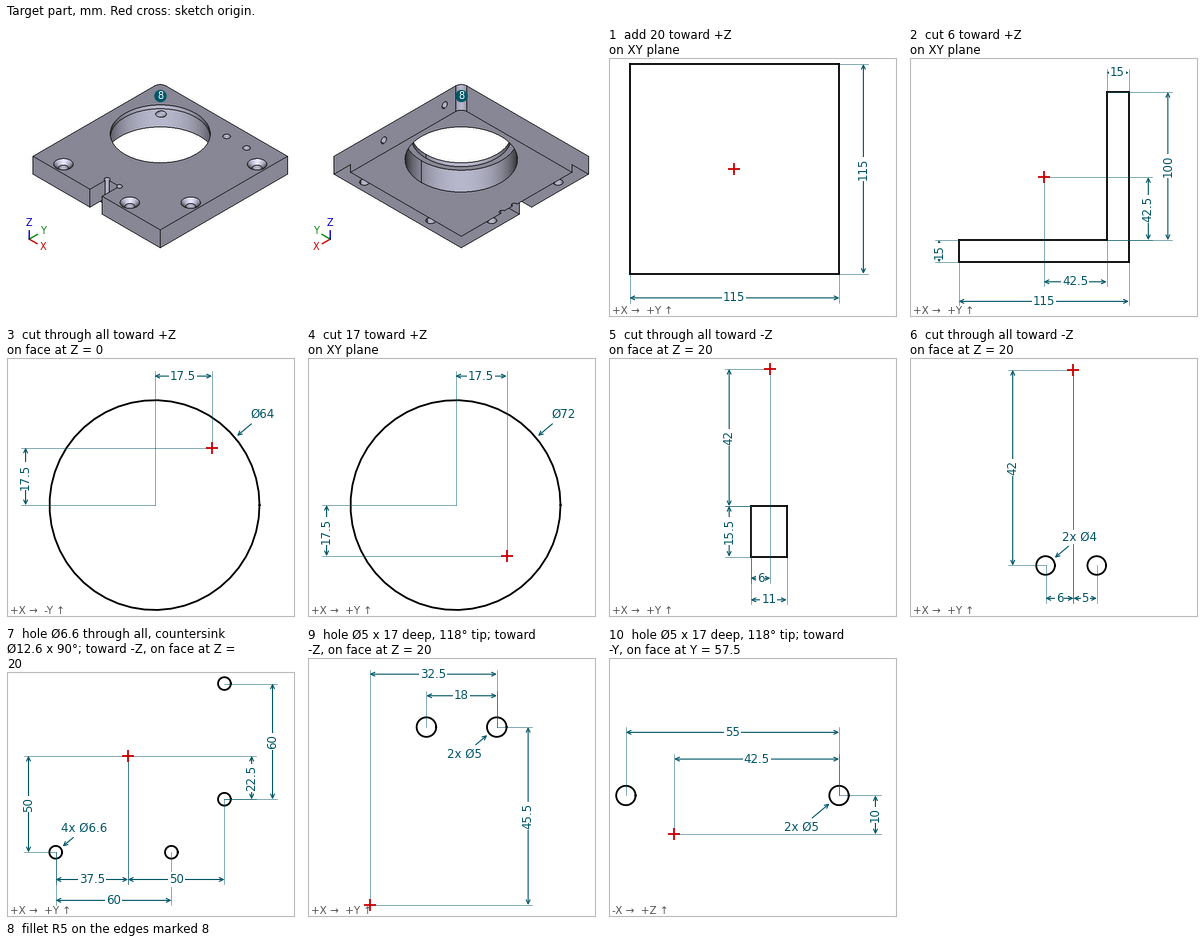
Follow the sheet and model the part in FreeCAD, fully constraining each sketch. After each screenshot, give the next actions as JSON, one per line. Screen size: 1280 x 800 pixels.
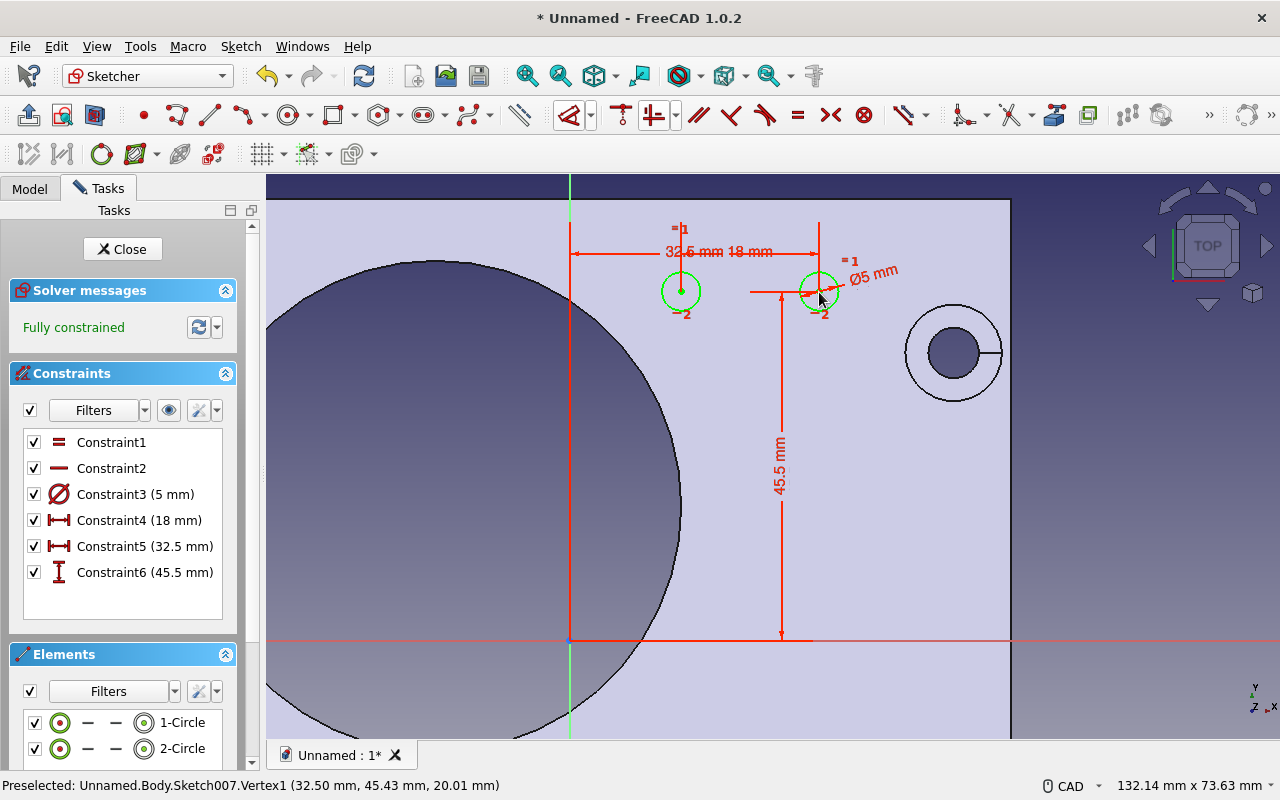
{"action": "left_click", "coordinate": [123, 249]}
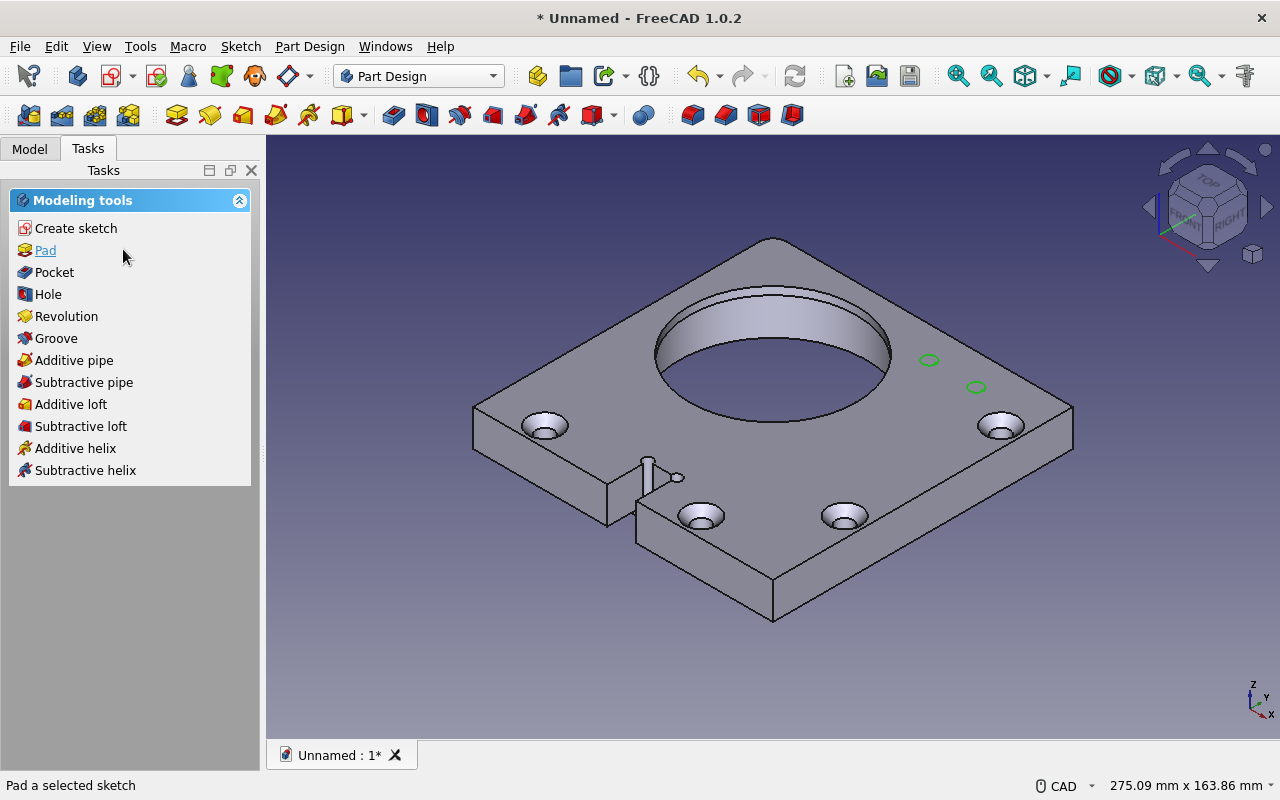
{"action": "left_click", "coordinate": [427, 116]}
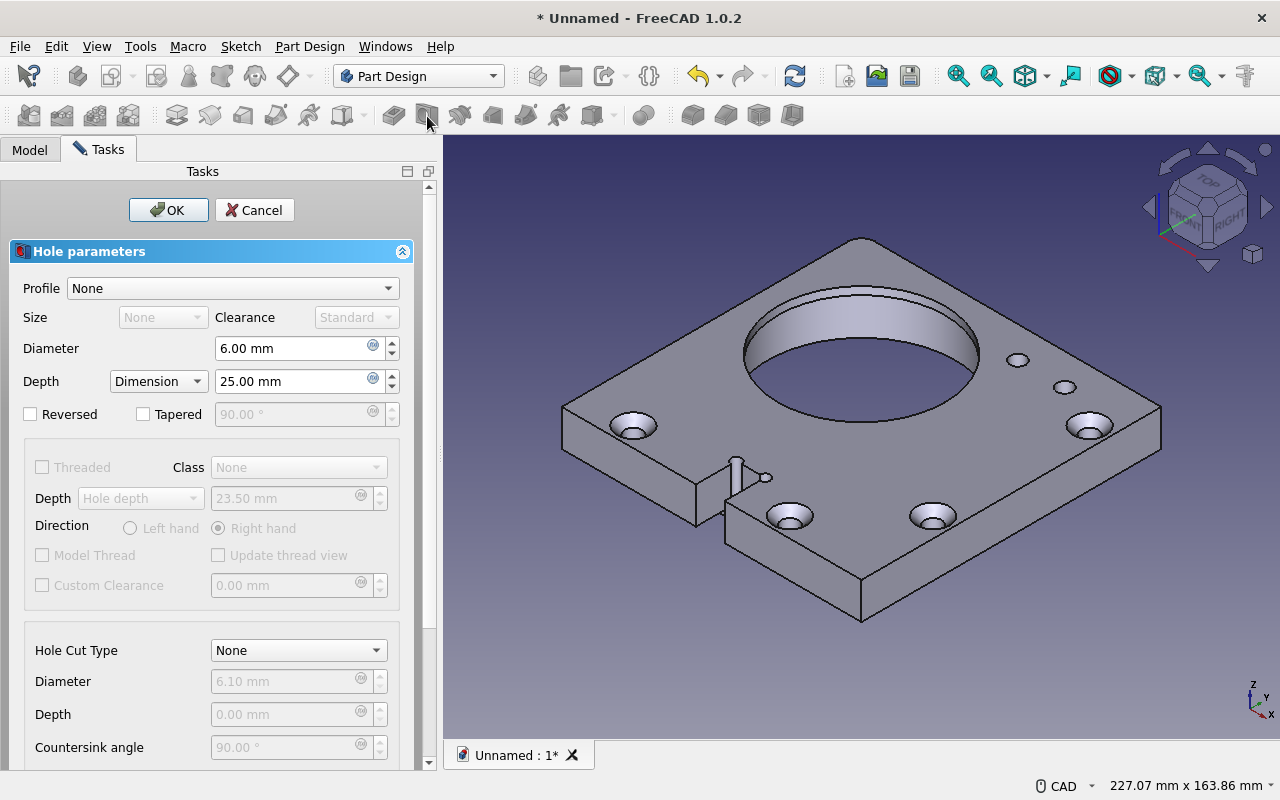
{"action": "triple_click", "coordinate": [300, 348]}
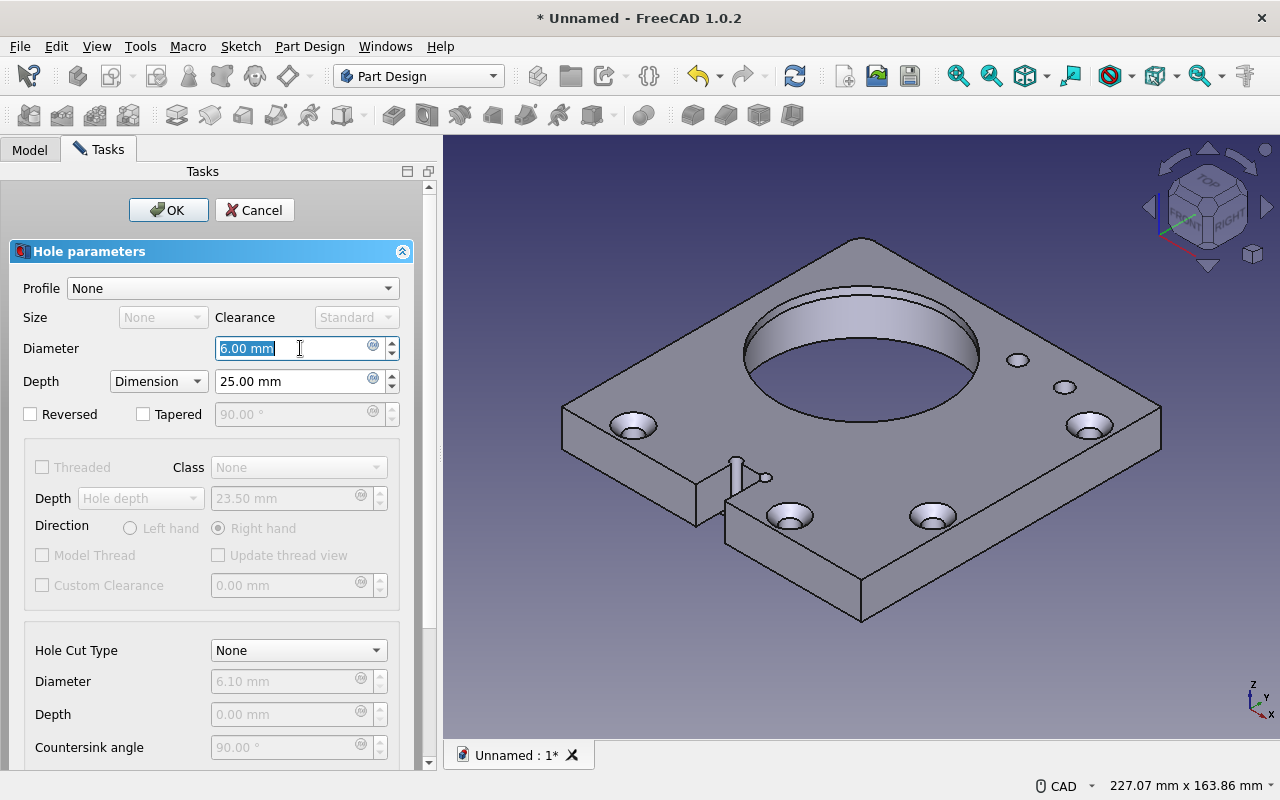
{"action": "type", "text": "5"}
{"action": "key", "text": "Tab"}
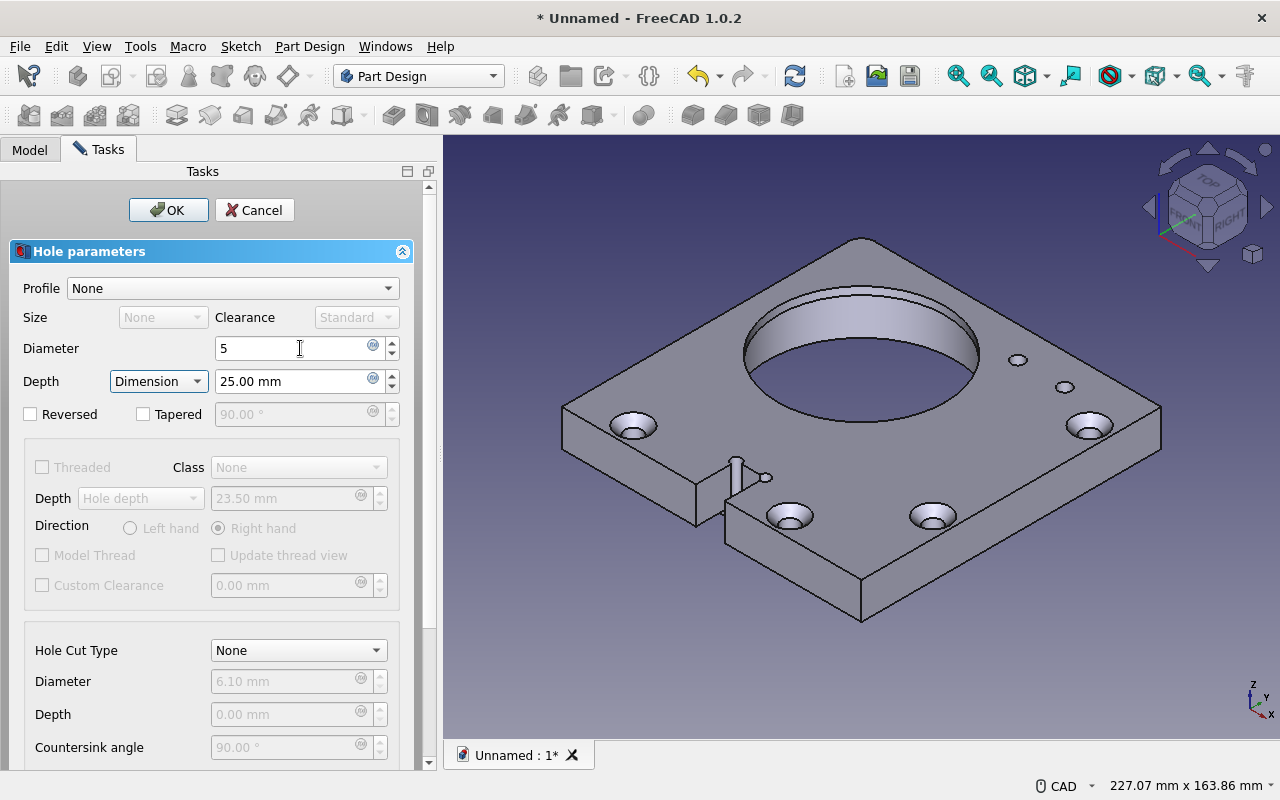
{"action": "triple_click", "coordinate": [300, 382]}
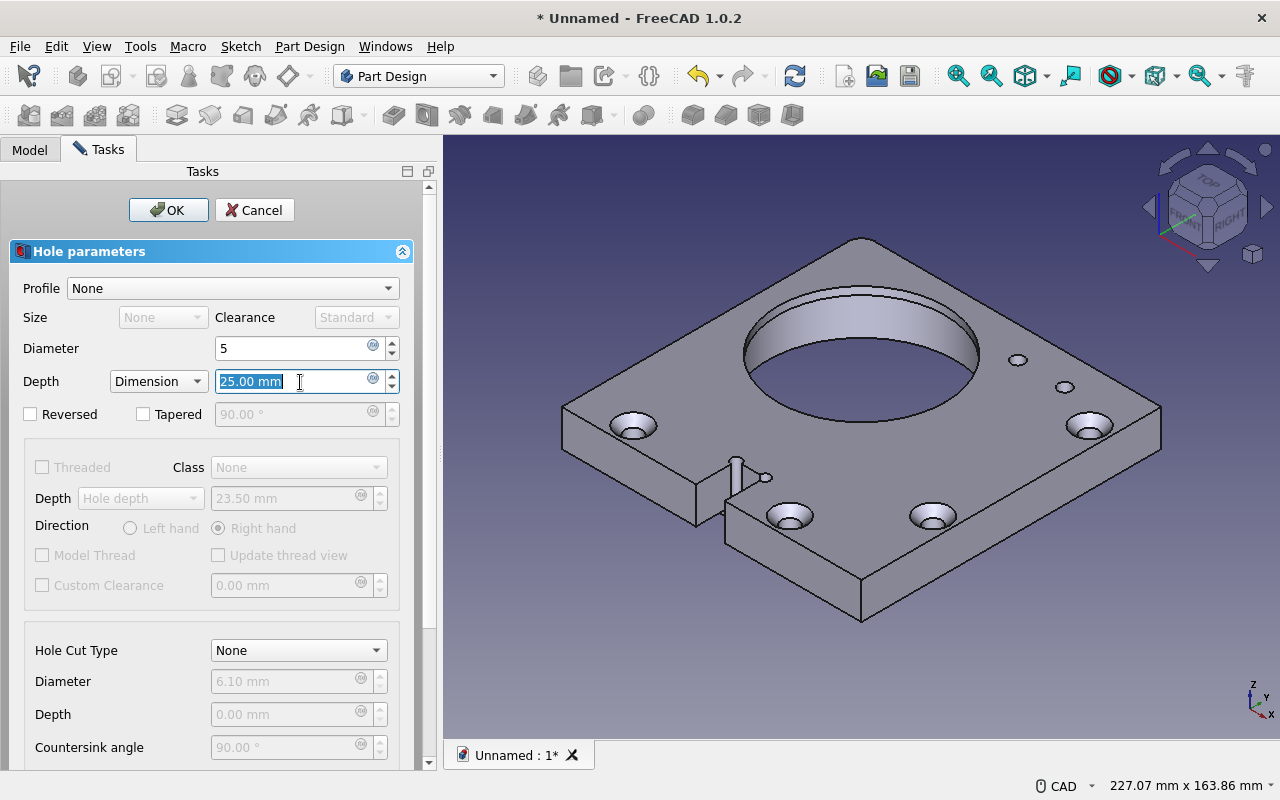
{"action": "type", "text": "17"}
{"action": "key", "text": "Tab"}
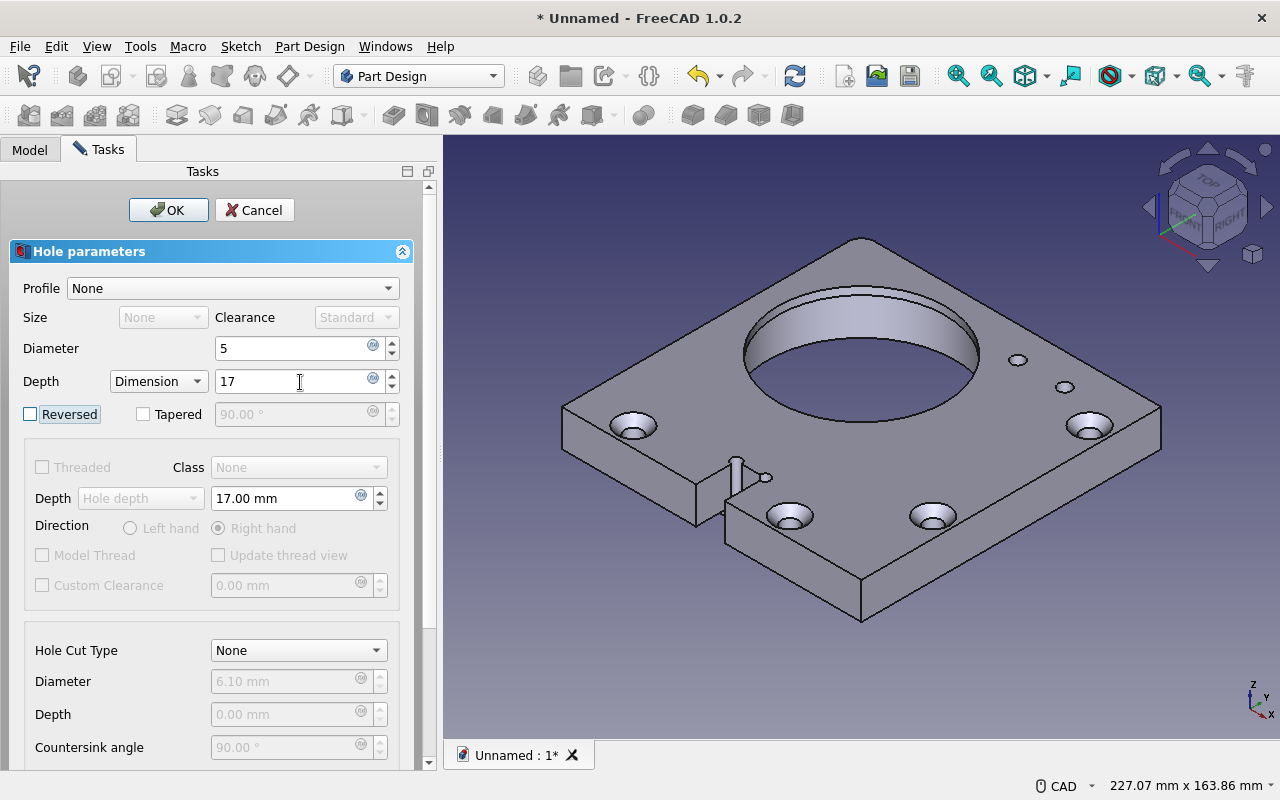
{"action": "left_click", "coordinate": [169, 210]}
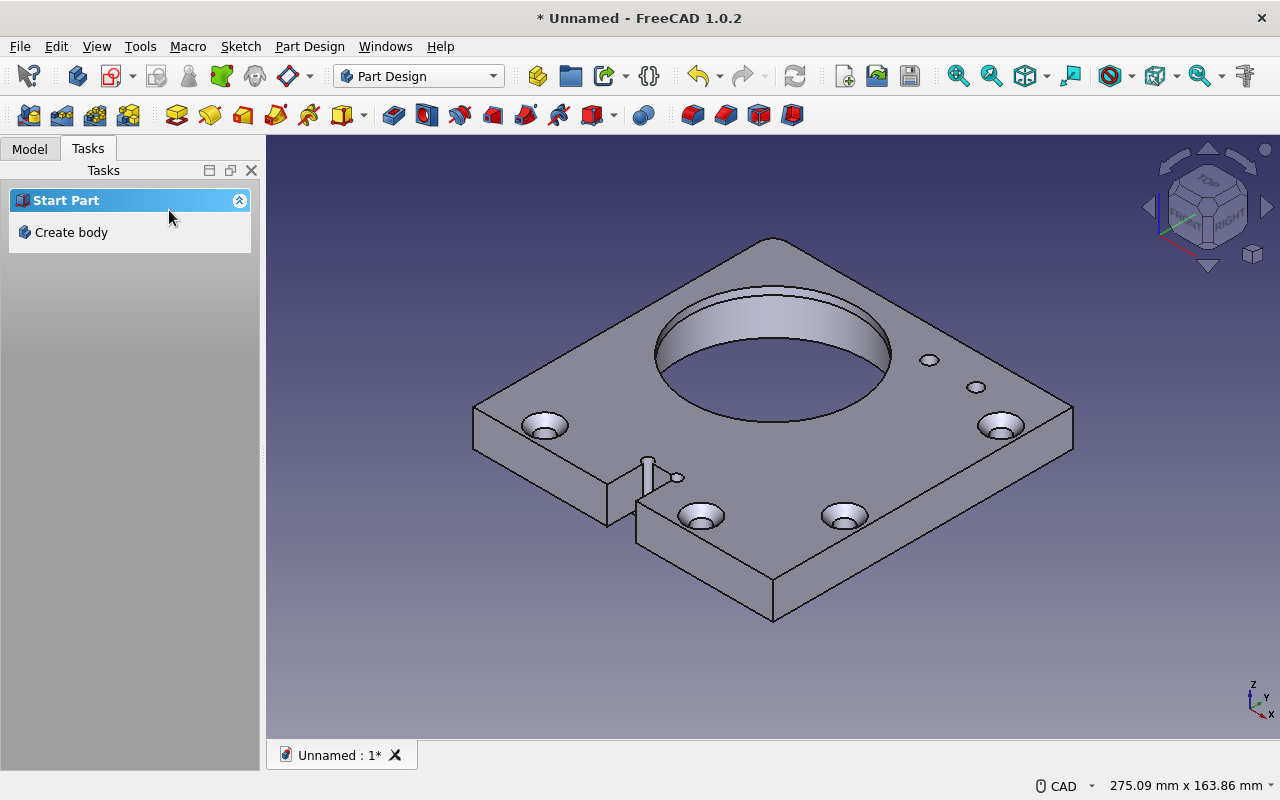
{"action": "key", "text": "4"}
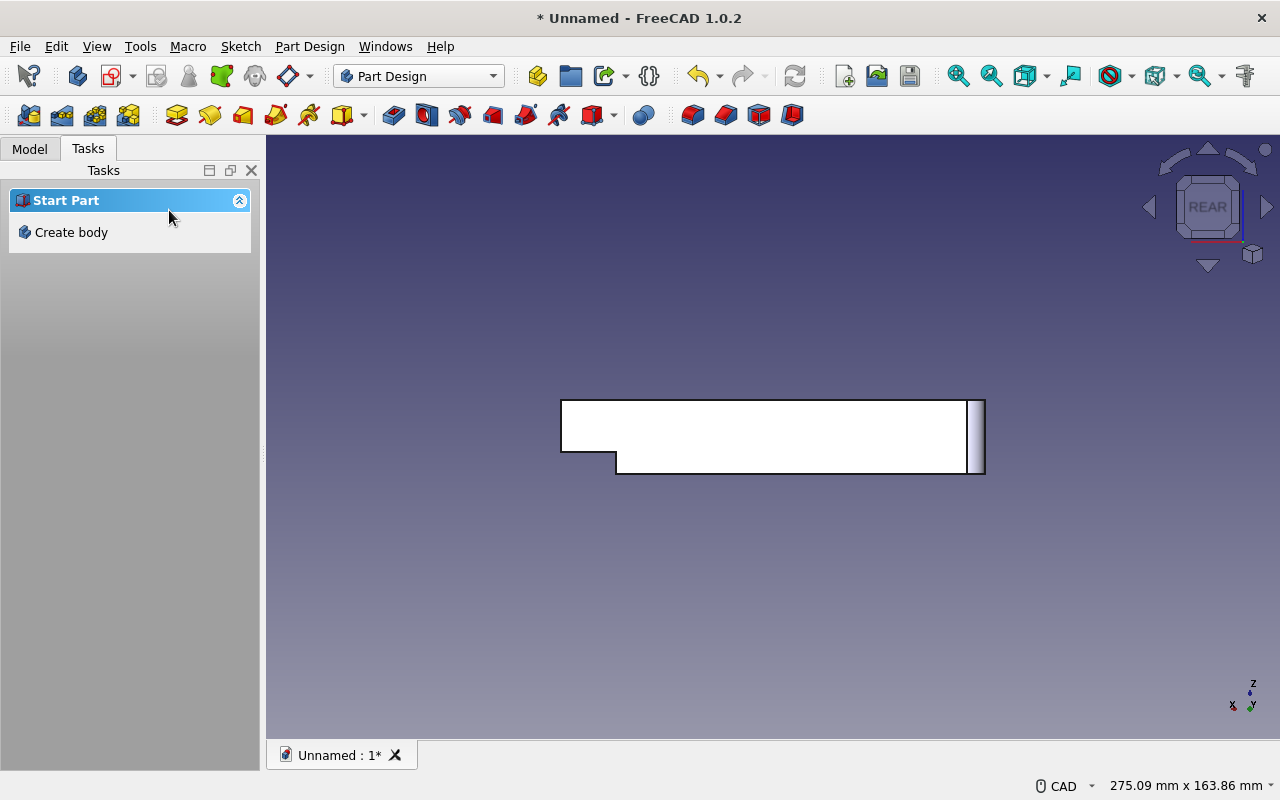
{"action": "key", "text": "v f"}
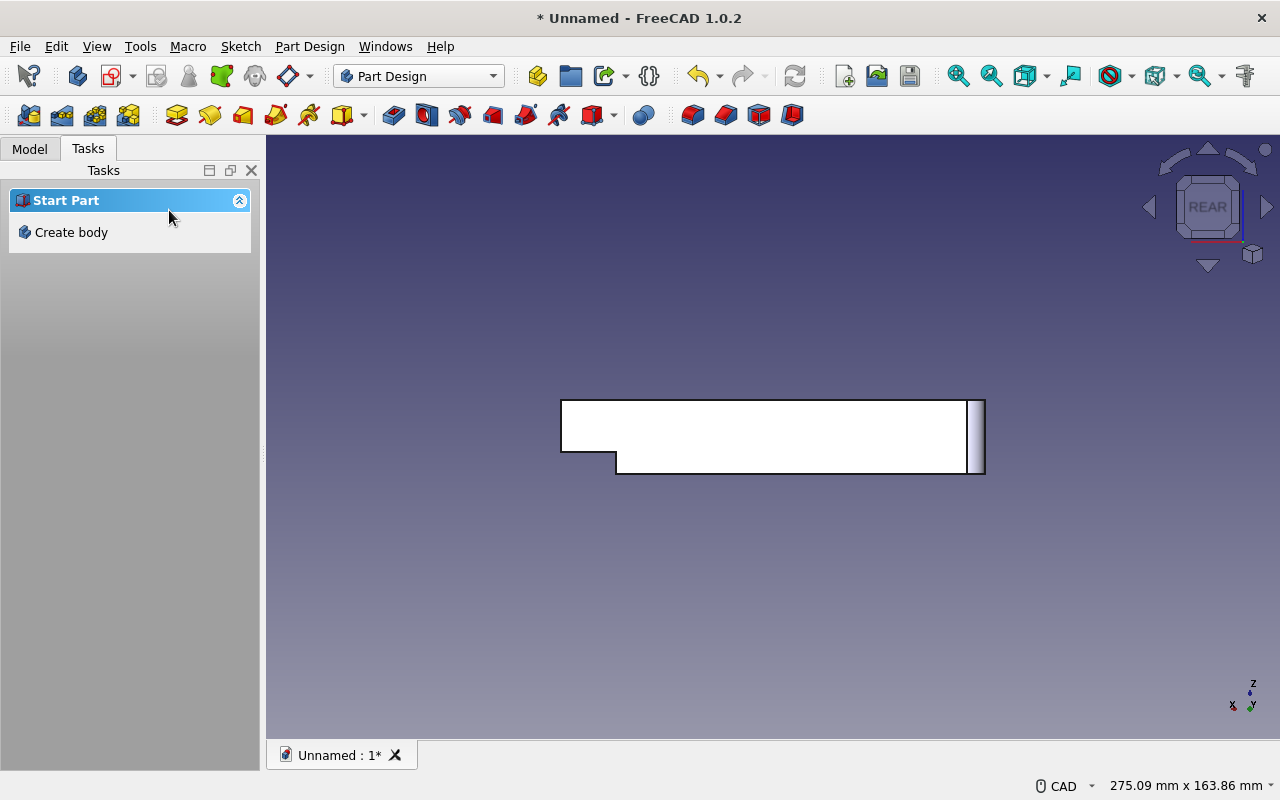
{"action": "left_click", "coordinate": [706, 436]}